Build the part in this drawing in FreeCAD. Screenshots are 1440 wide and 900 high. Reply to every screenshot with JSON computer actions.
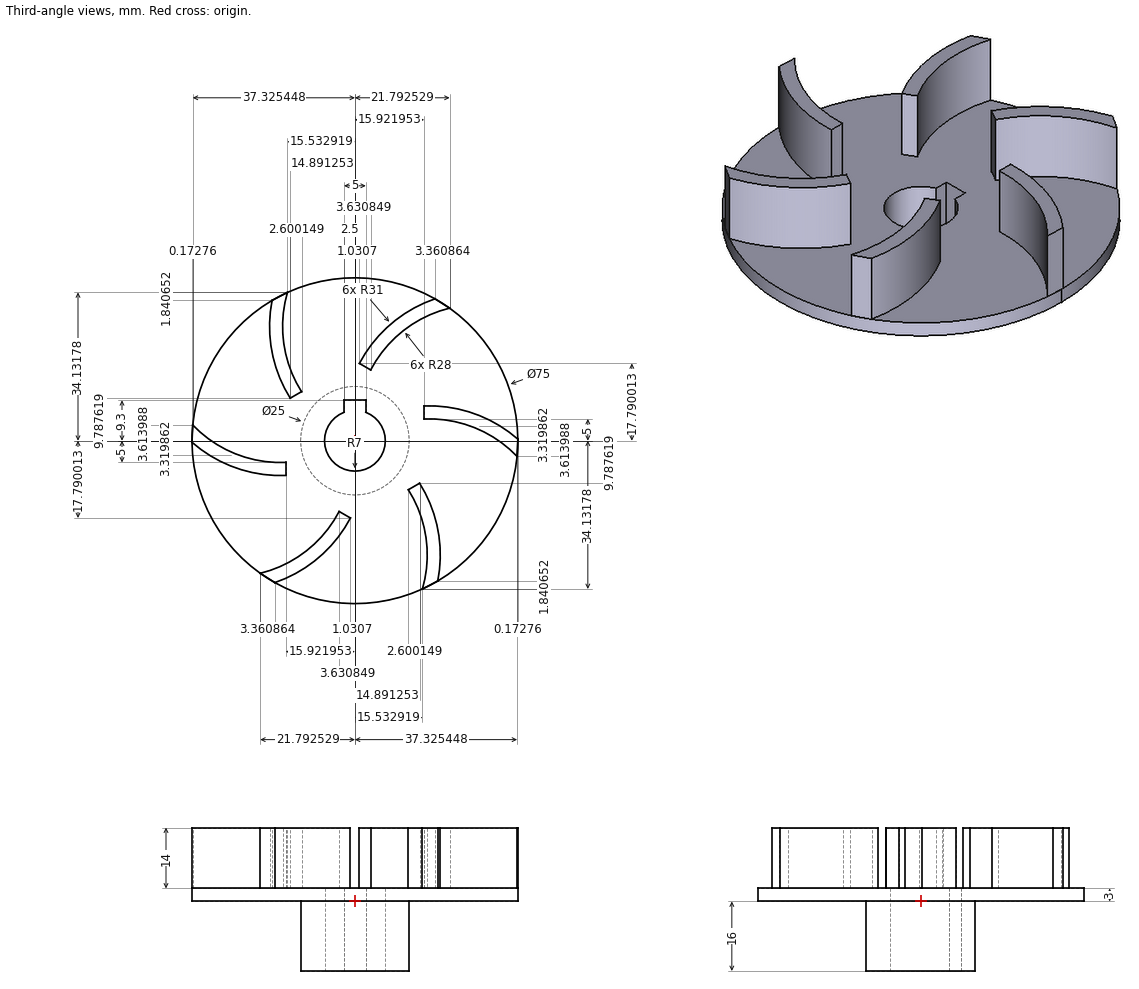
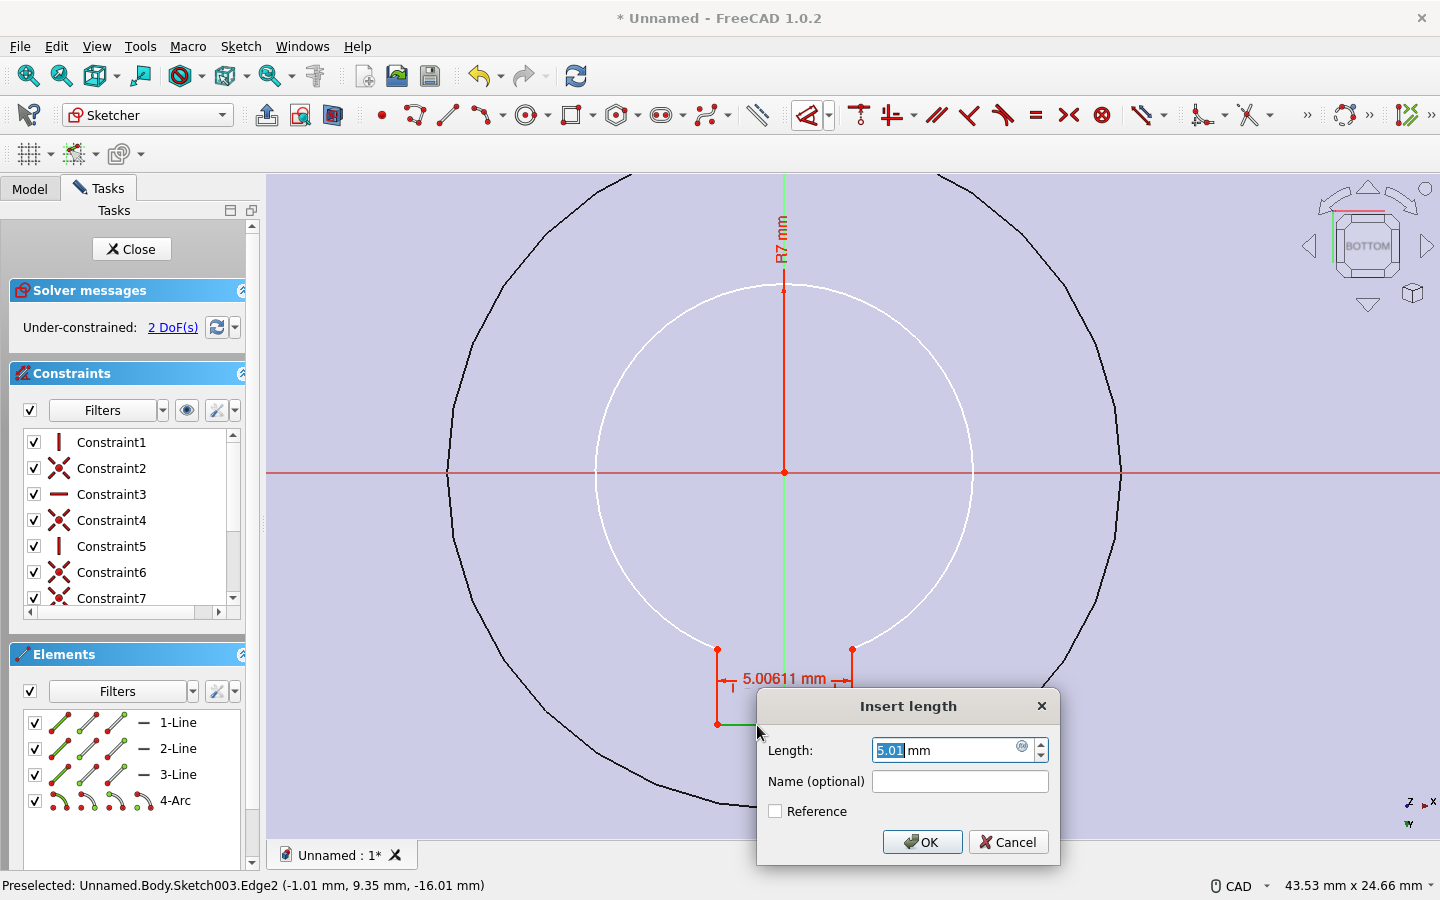
{"action": "type", "text": "5"}
{"action": "key", "text": "Return"}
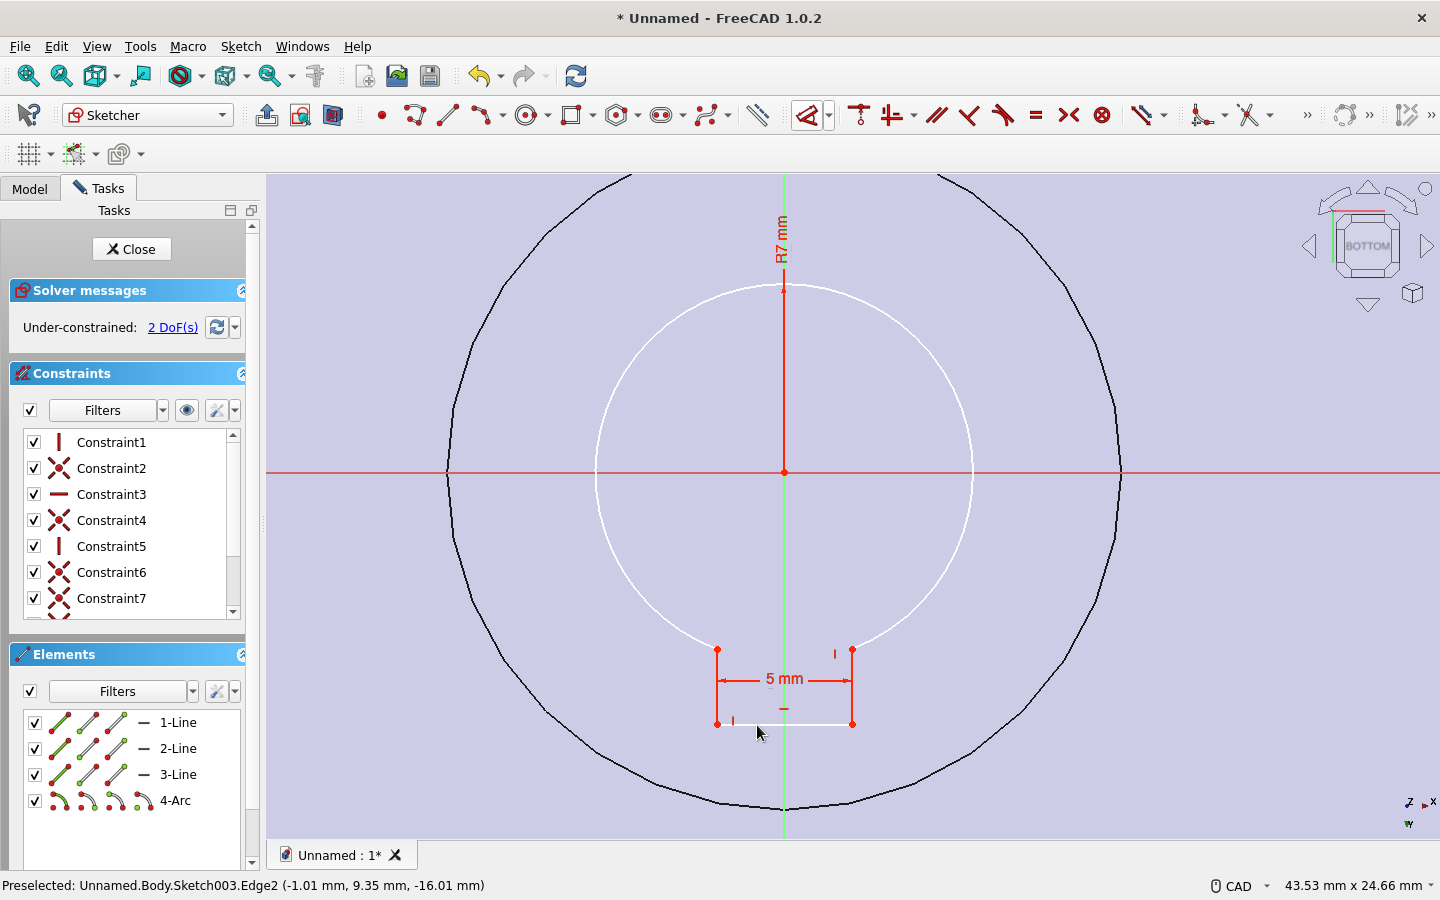
{"action": "left_click", "coordinate": [717, 649]}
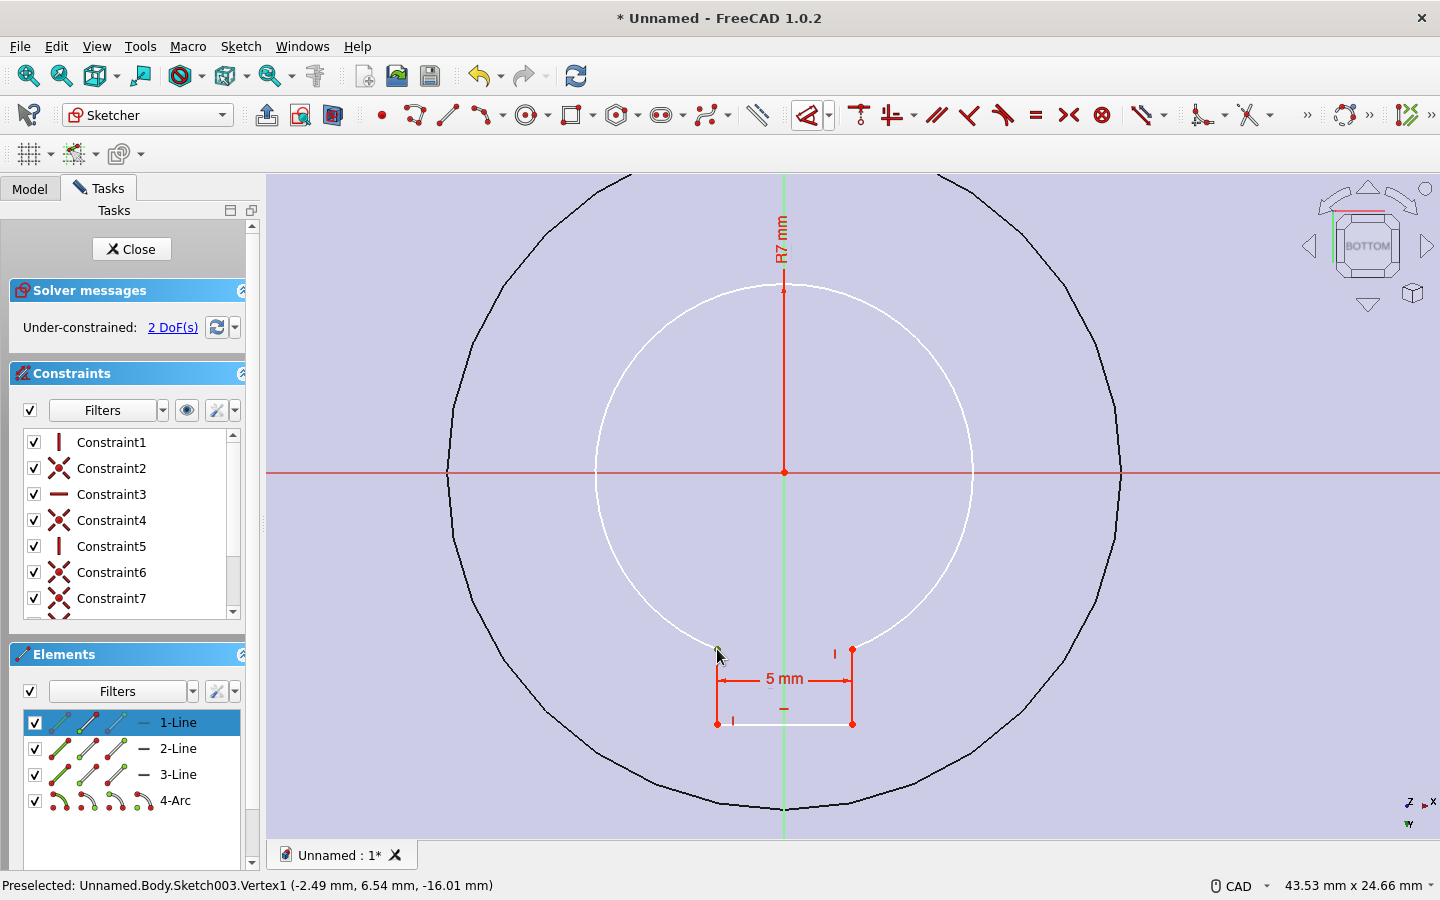
{"action": "left_click", "coordinate": [828, 116]}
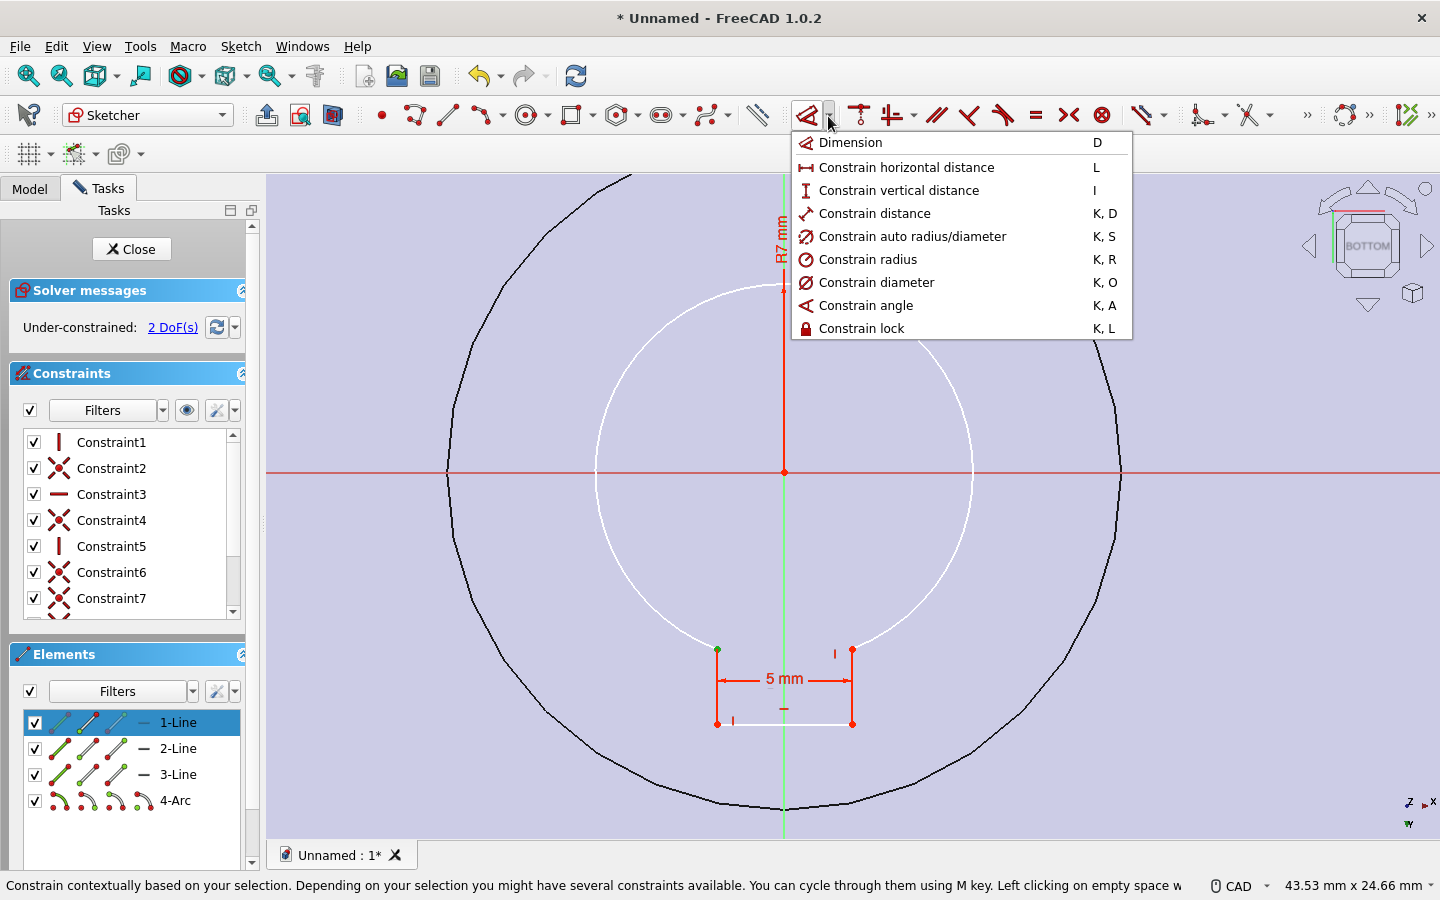
{"action": "left_click", "coordinate": [962, 168]}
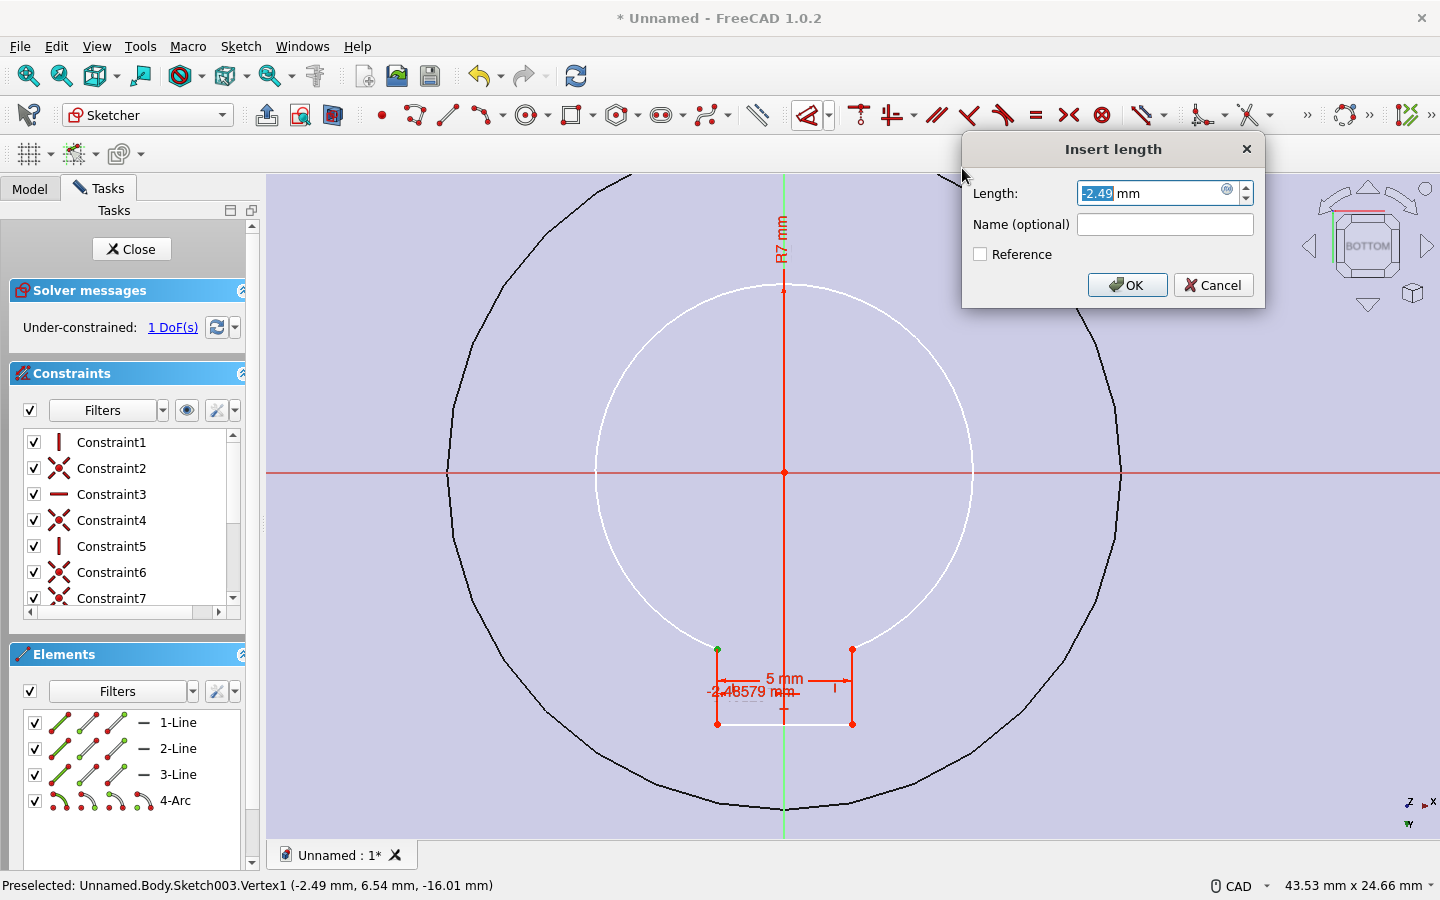
{"action": "type", "text": "-2.5"}
{"action": "key", "text": "Return"}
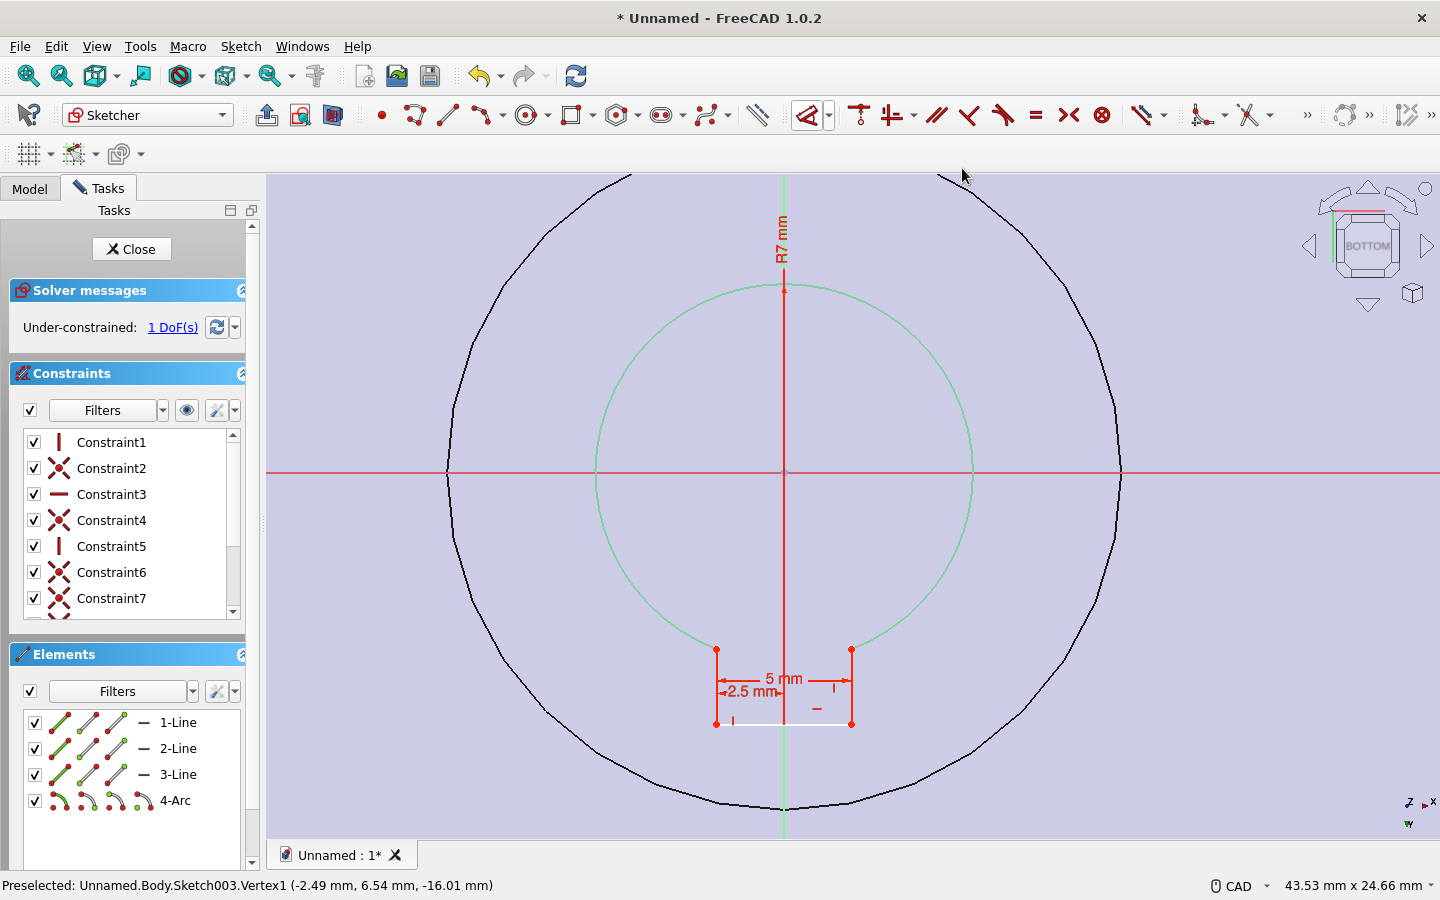
{"action": "left_click", "coordinate": [717, 725]}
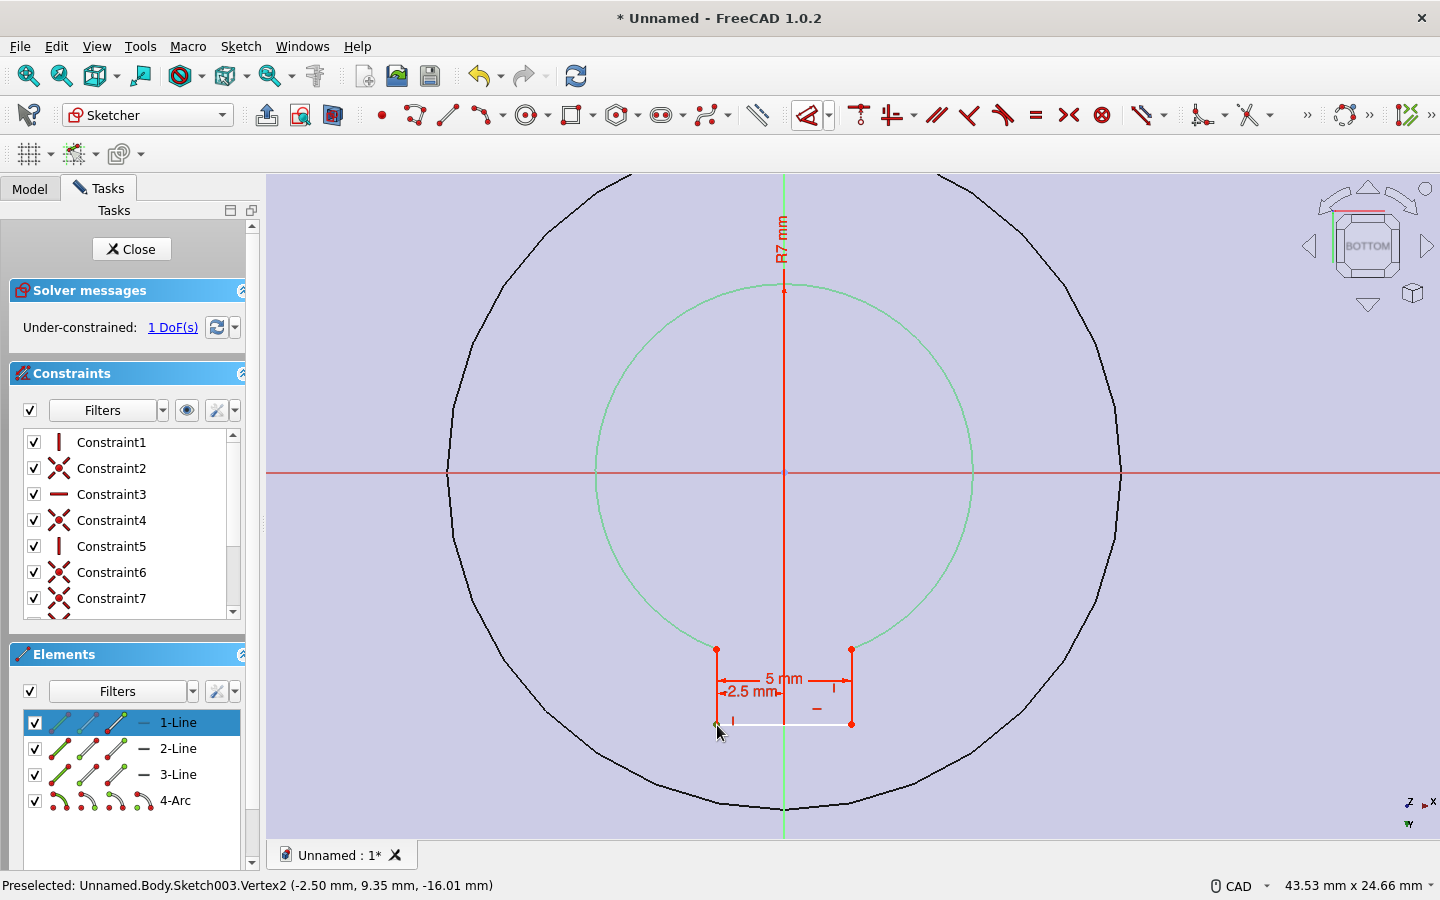
{"action": "key", "text": "i"}